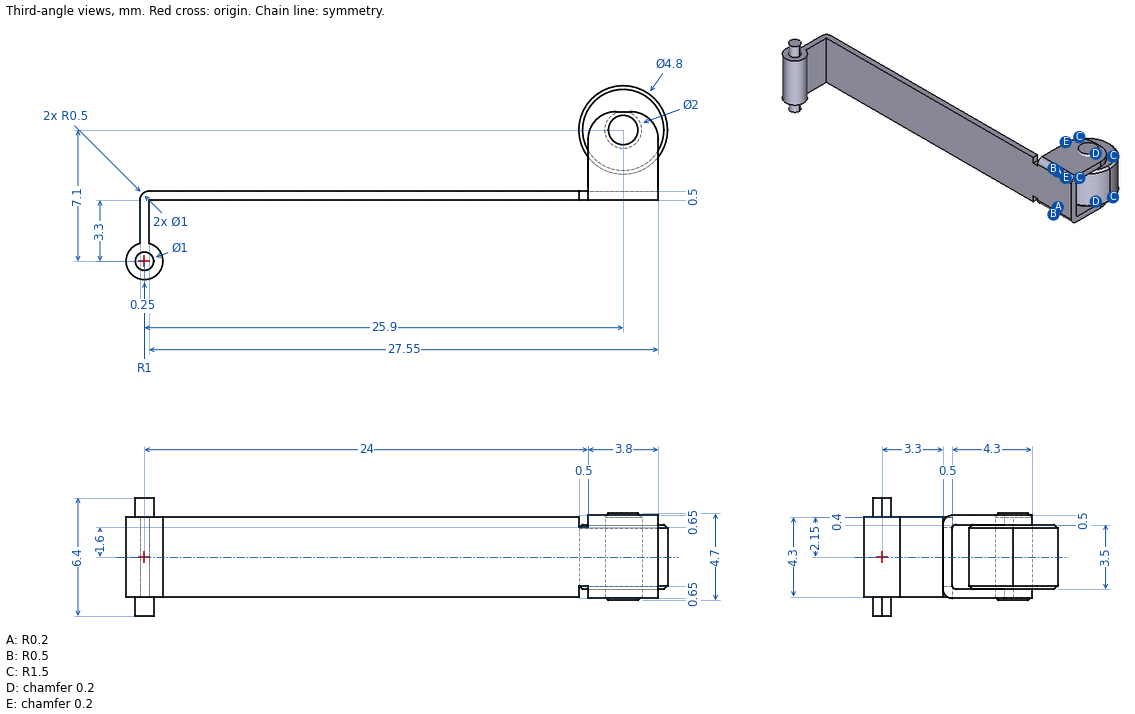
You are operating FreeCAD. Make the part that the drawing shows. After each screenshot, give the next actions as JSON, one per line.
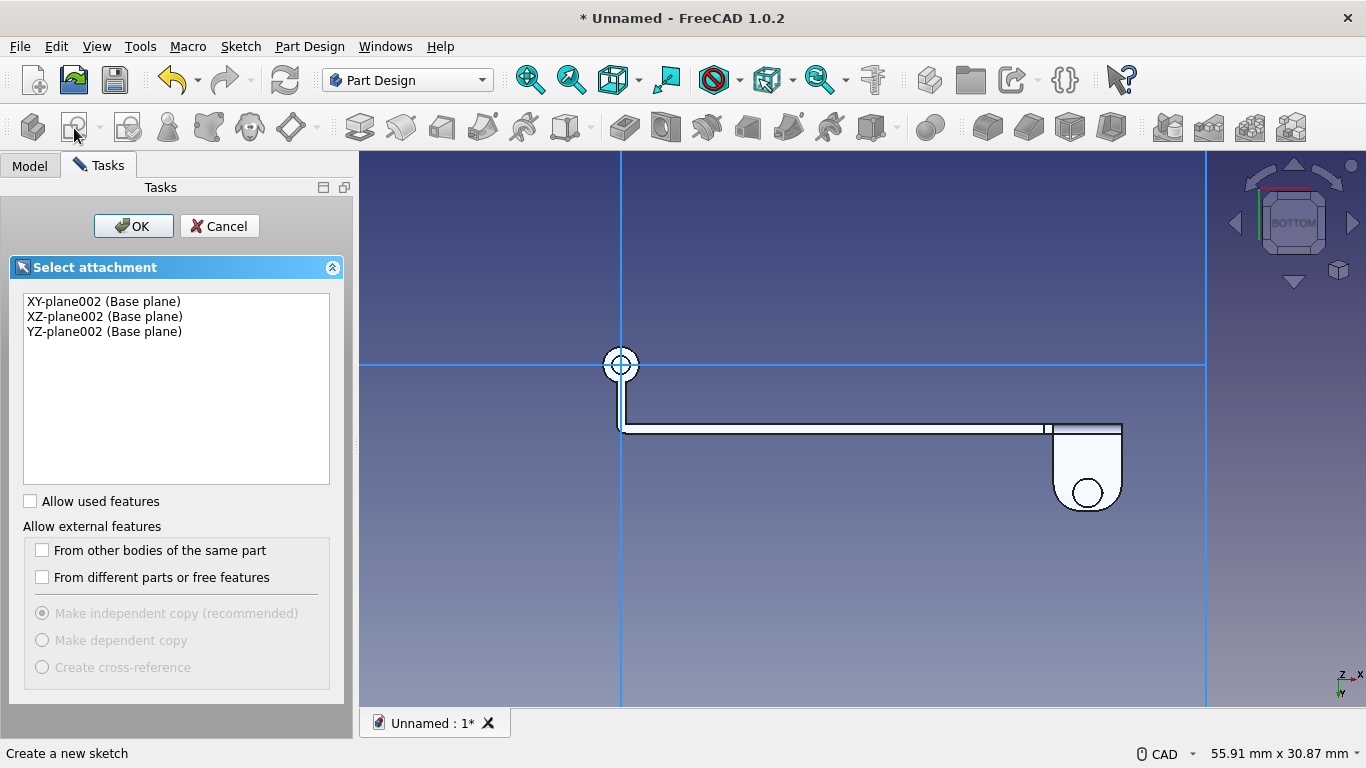
{"action": "left_click", "coordinate": [84, 302]}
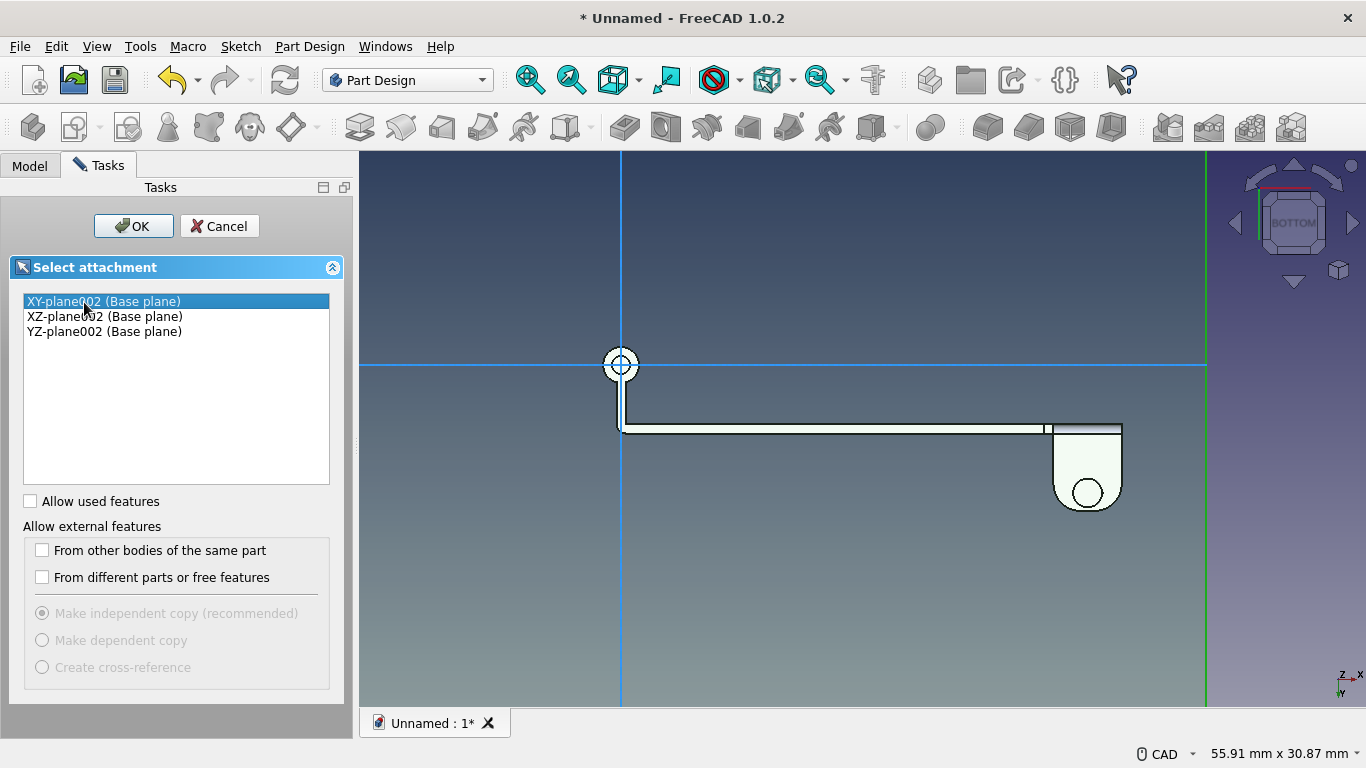
{"action": "left_click", "coordinate": [134, 226]}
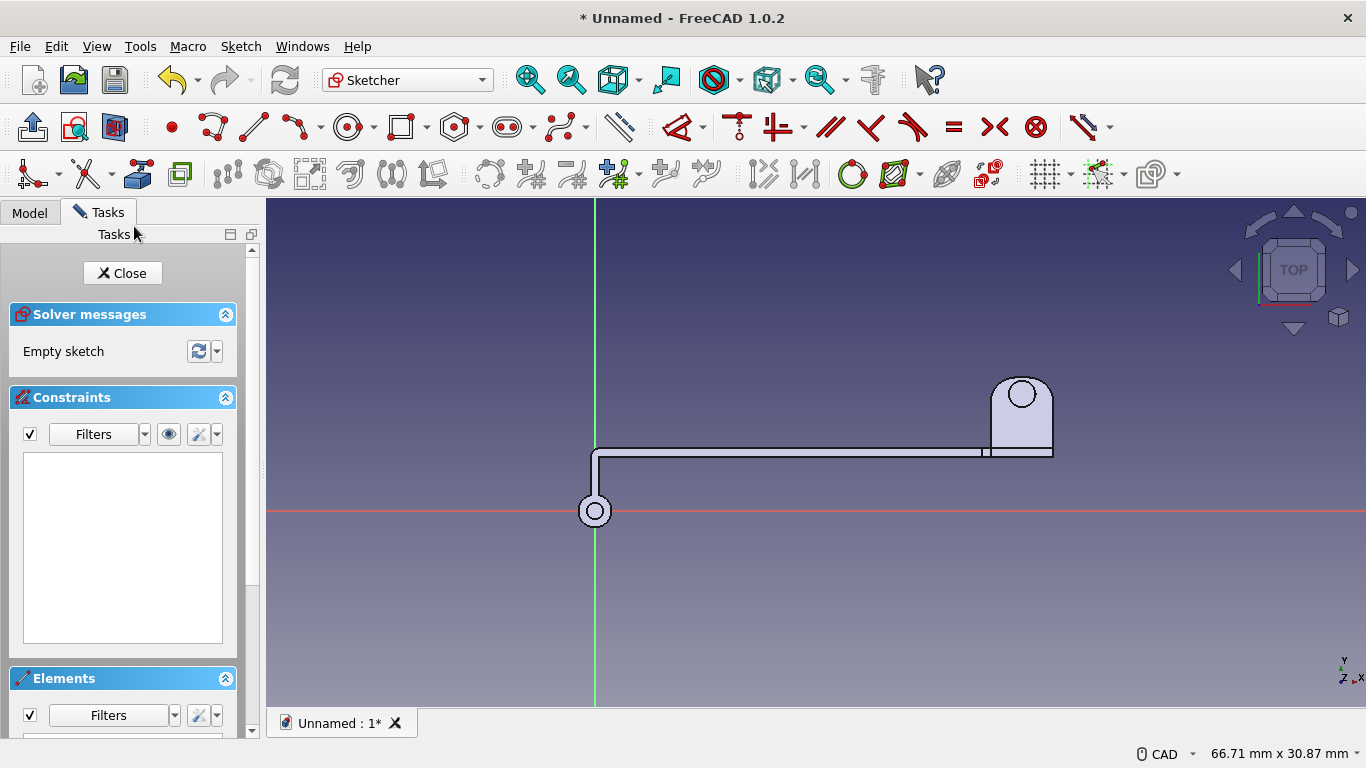
{"action": "scroll", "coordinate": [1112, 375], "scroll_direction": "up", "scroll_amount": 7}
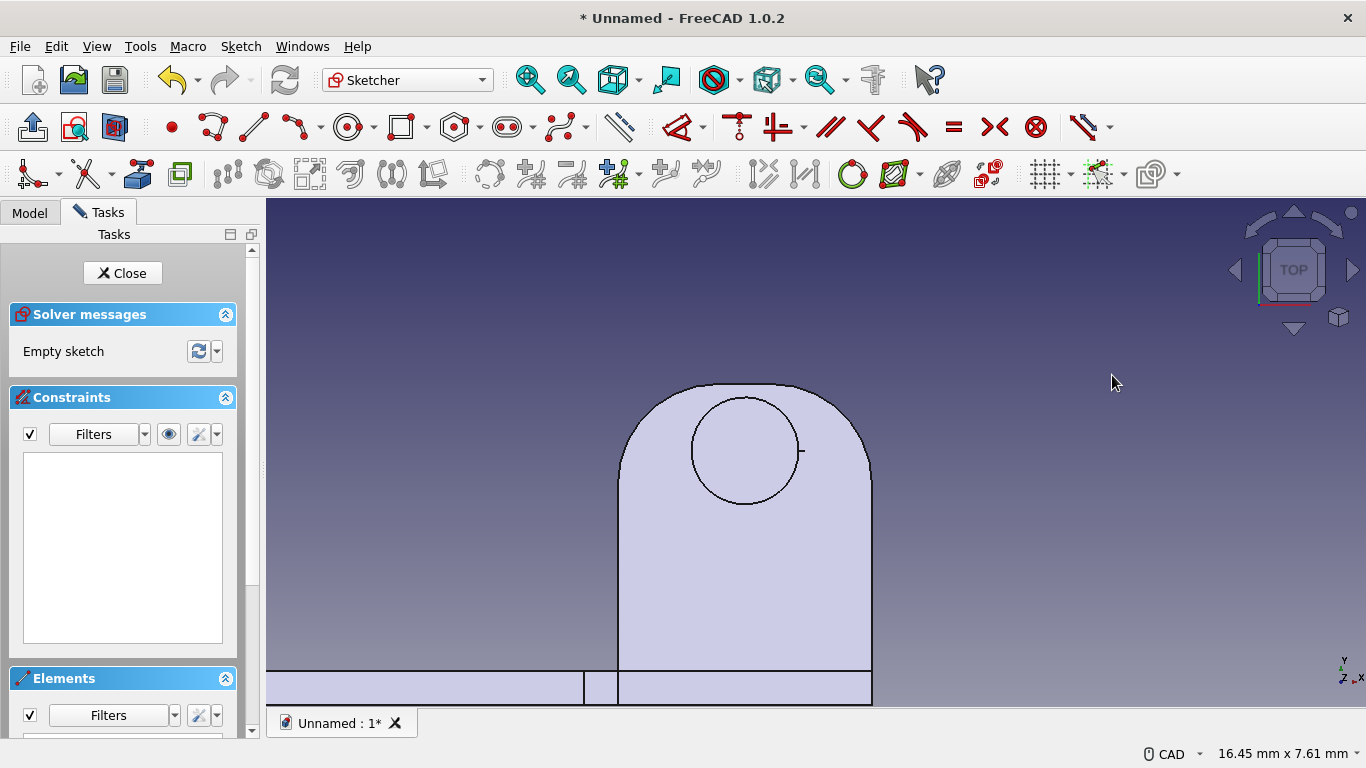
{"action": "left_click", "coordinate": [348, 128]}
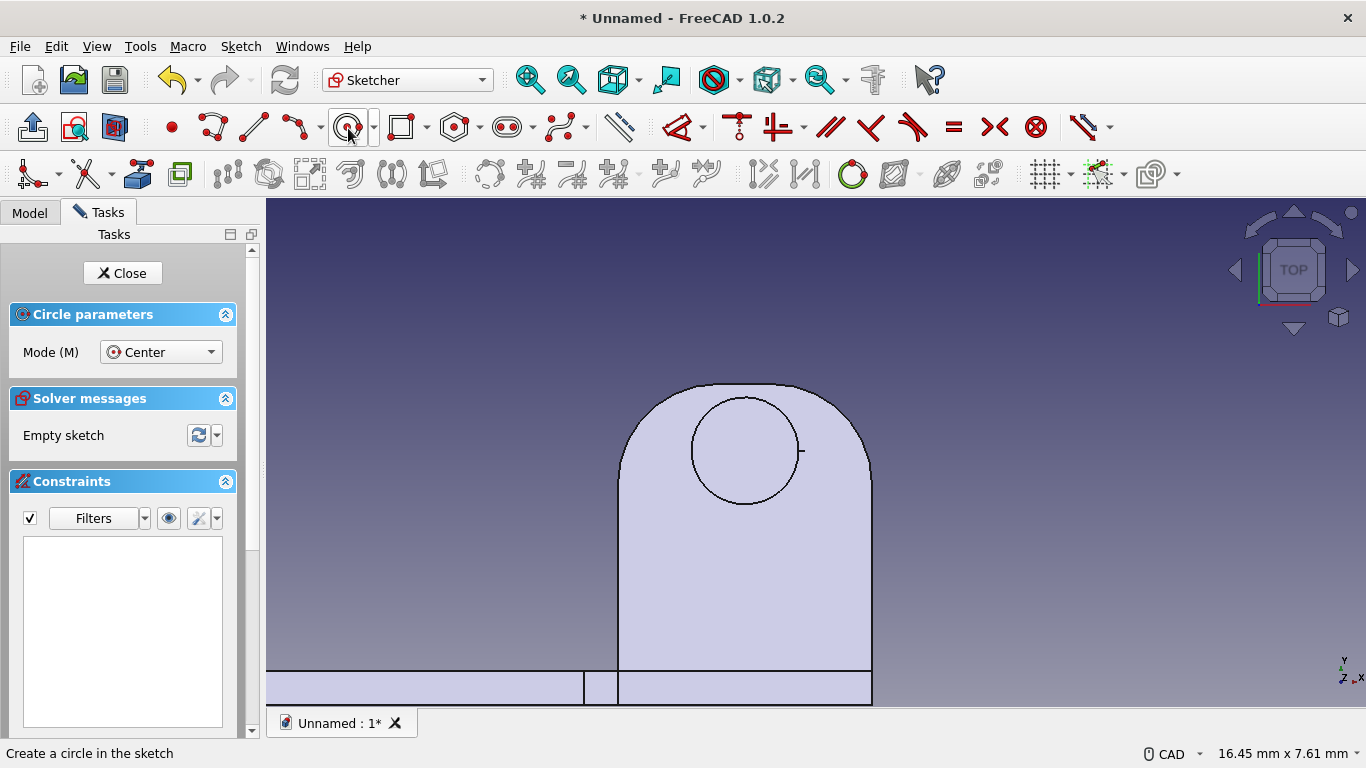
{"action": "left_click", "coordinate": [745, 451]}
{"action": "mouse_move", "coordinate": [858, 337]}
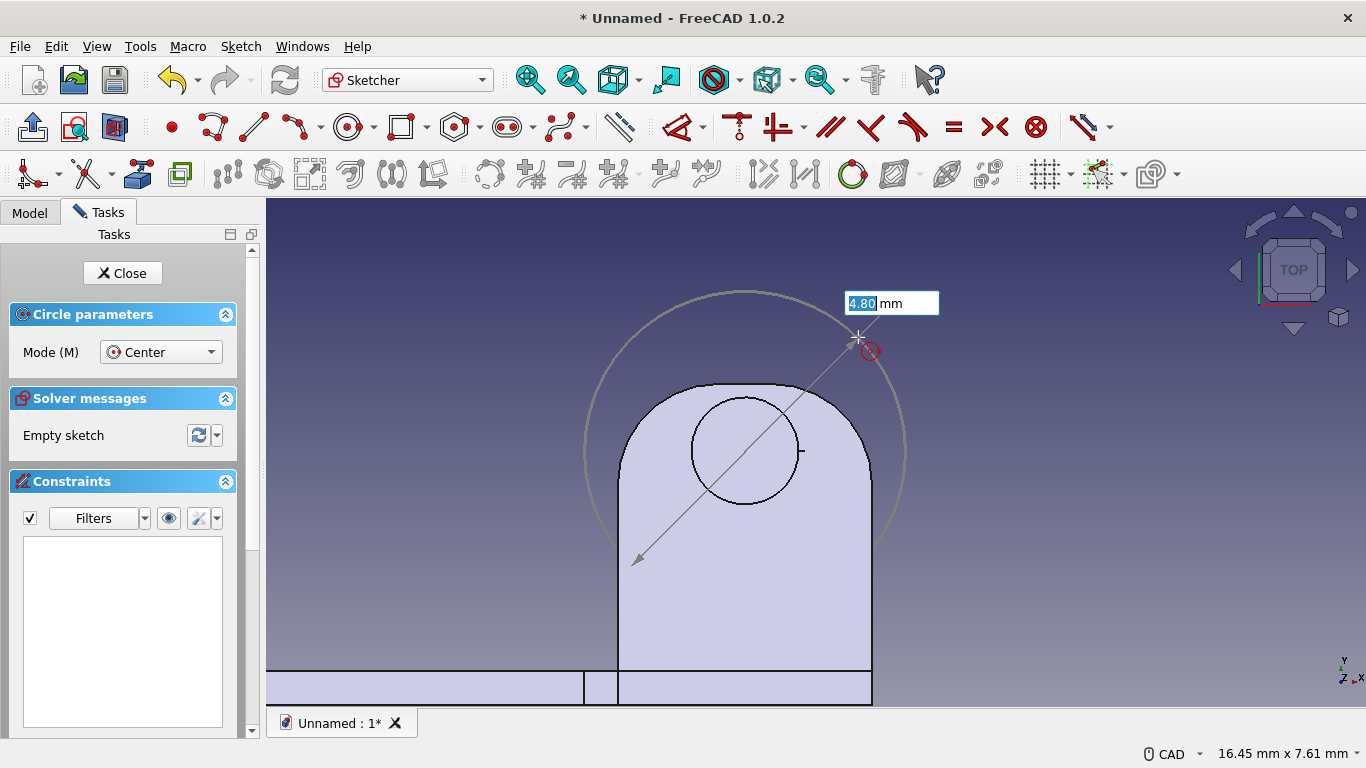
{"action": "type", "text": "4.8"}
{"action": "key", "text": "Return"}
{"action": "key", "text": "Escape"}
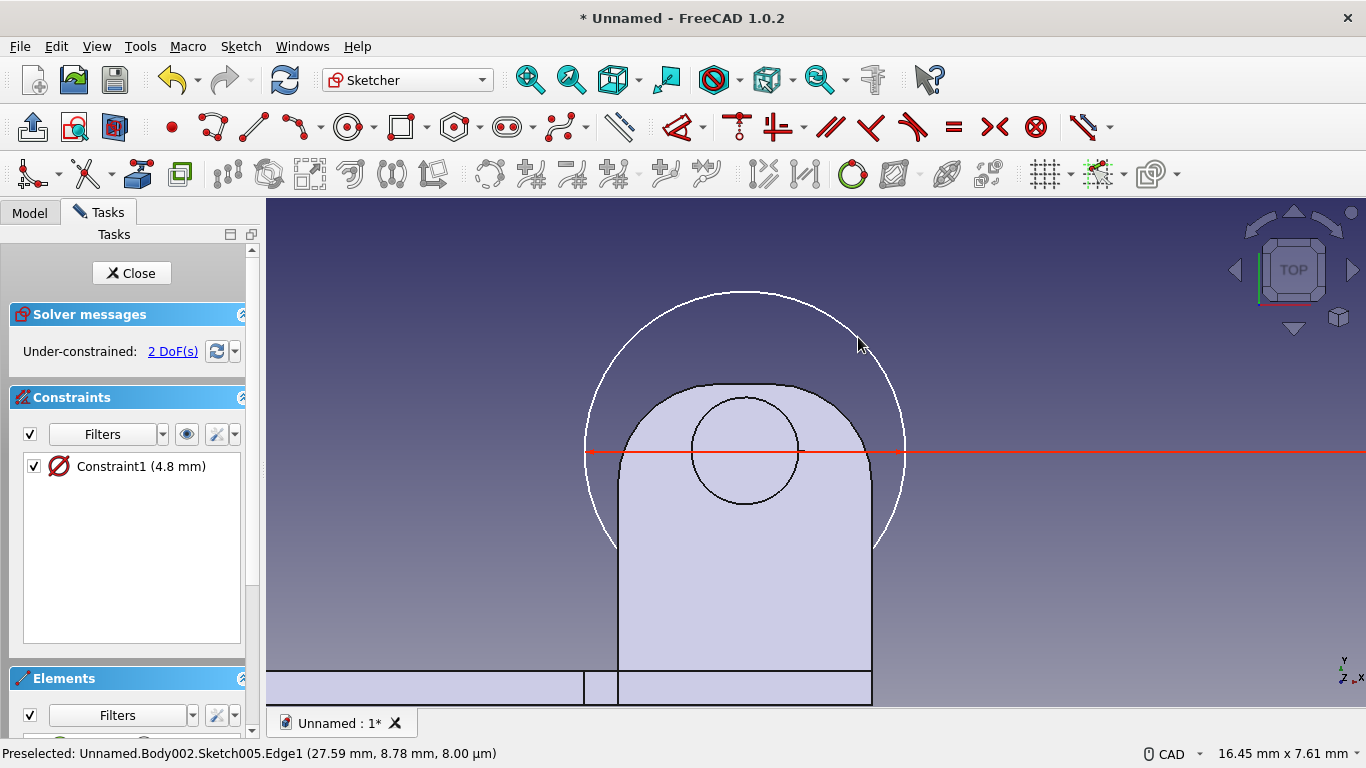
{"action": "key", "text": "d"}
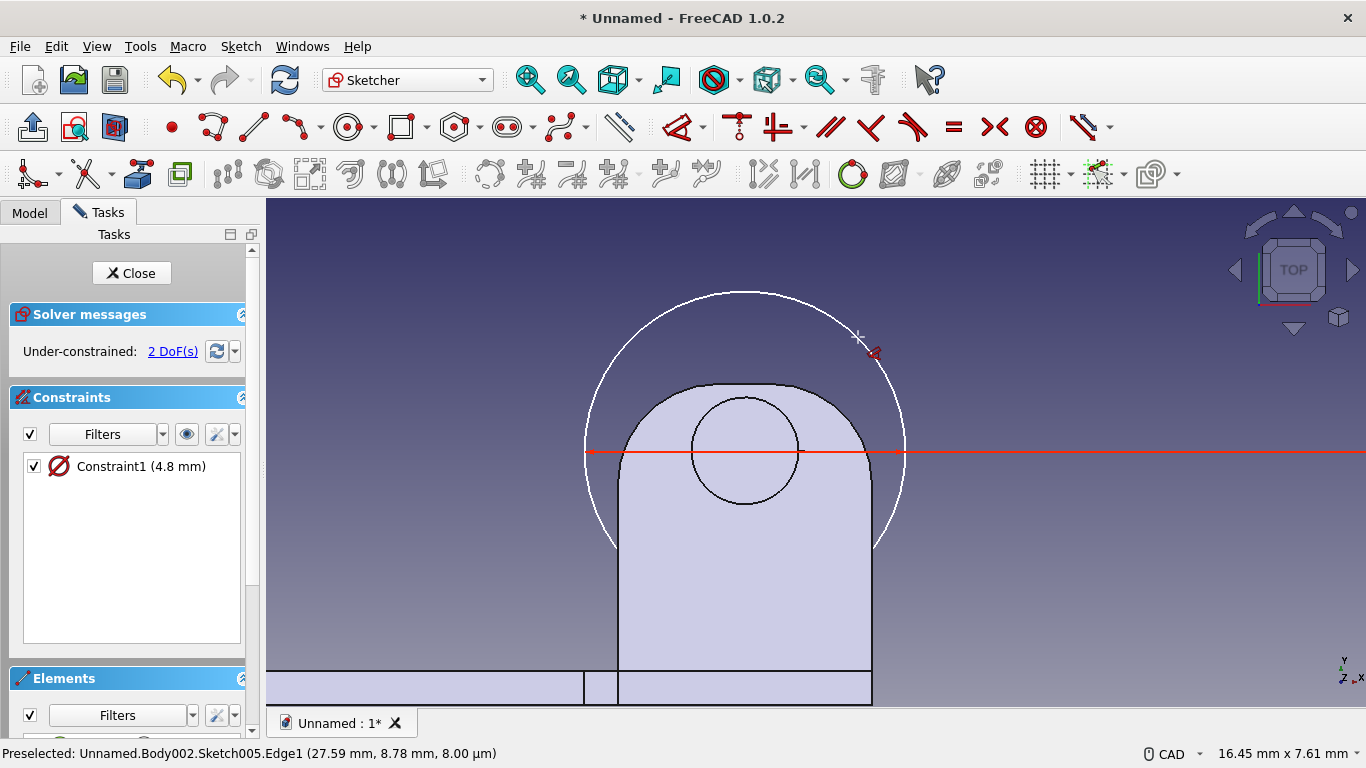
{"action": "left_click", "coordinate": [745, 452]}
{"action": "left_click", "coordinate": [779, 565]}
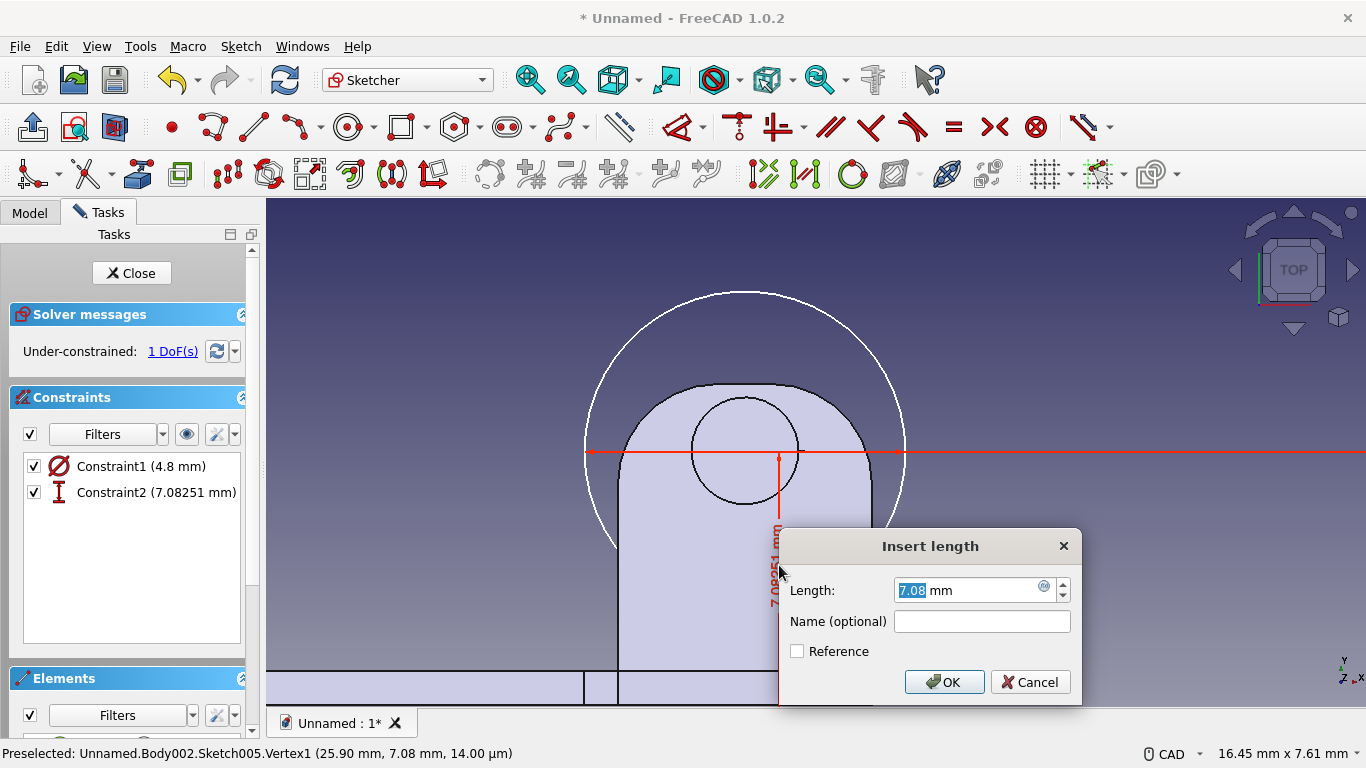
{"action": "type", "text": "7.1"}
{"action": "key", "text": "Return"}